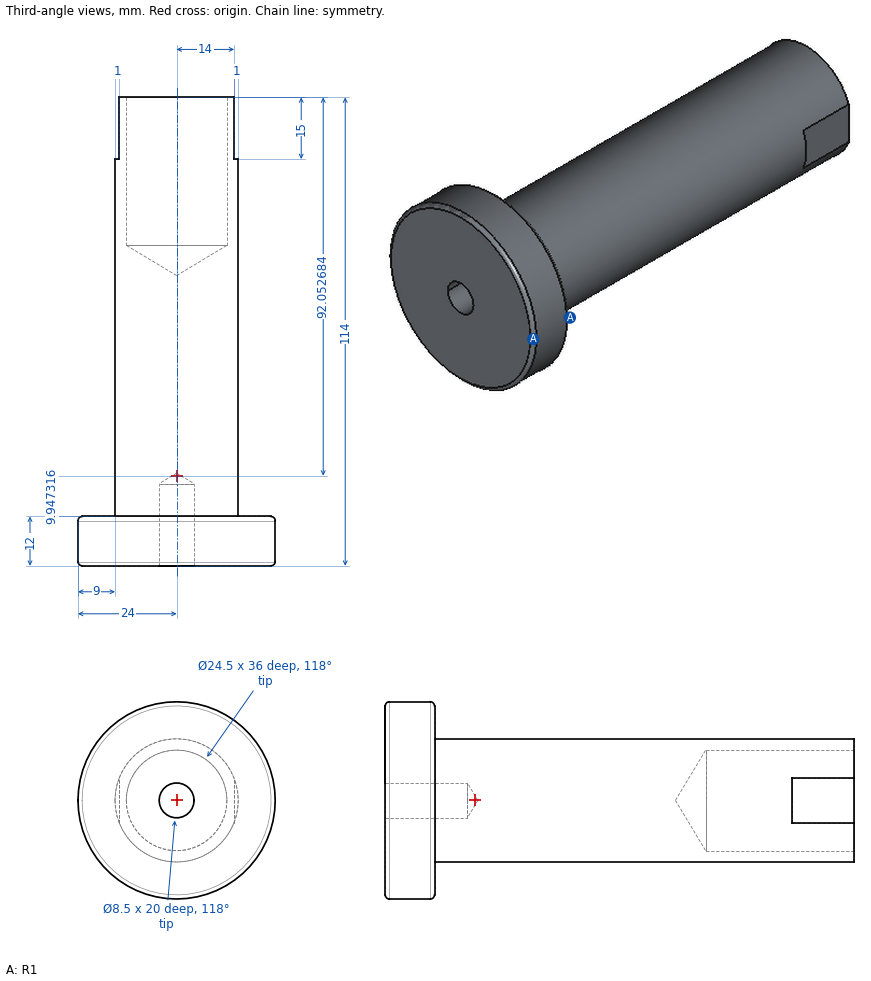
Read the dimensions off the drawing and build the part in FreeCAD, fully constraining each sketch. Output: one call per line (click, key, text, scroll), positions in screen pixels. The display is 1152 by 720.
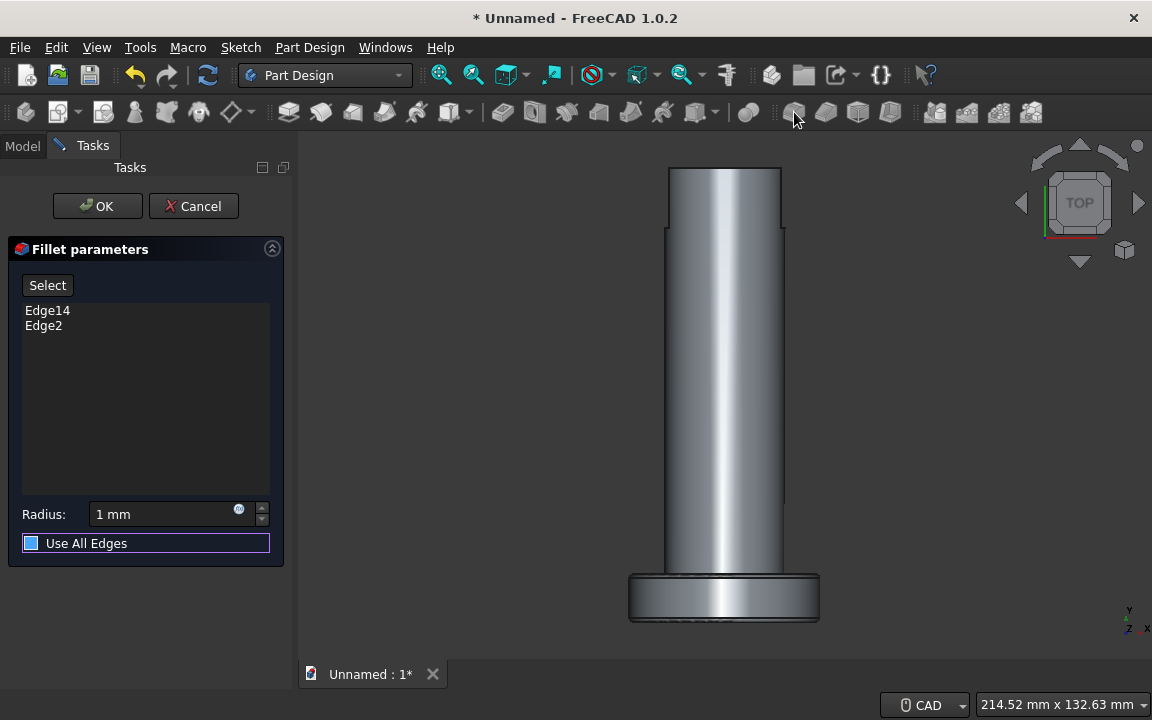
click(98, 206)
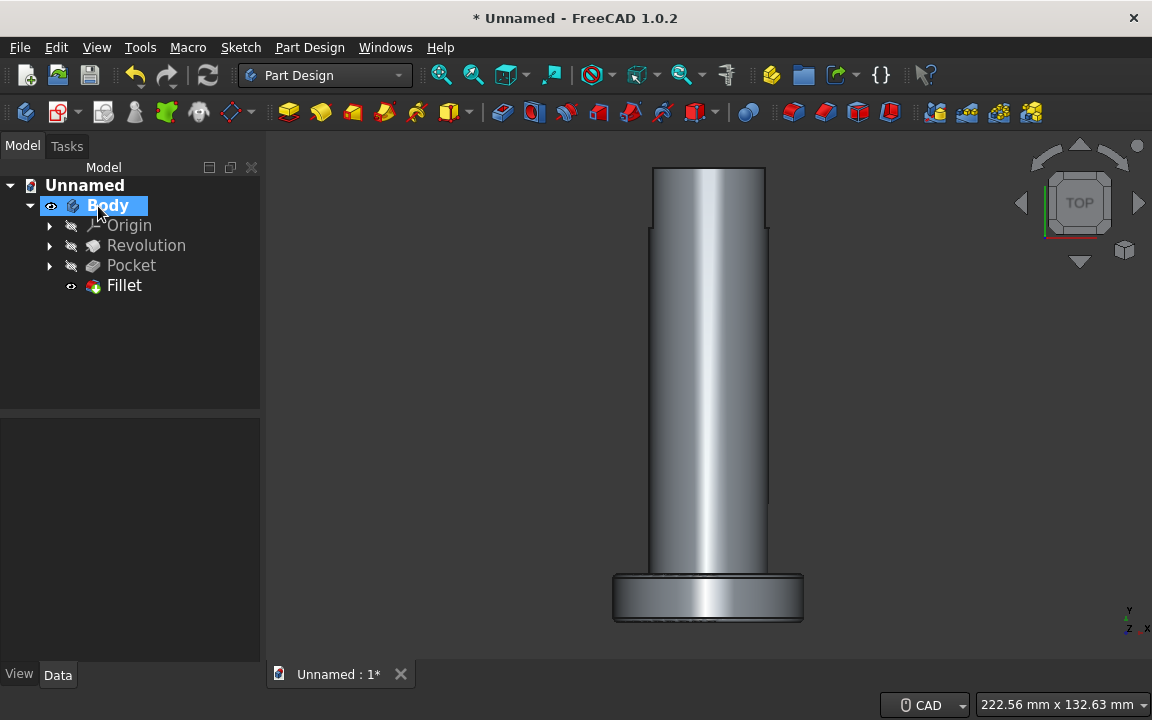
key(4)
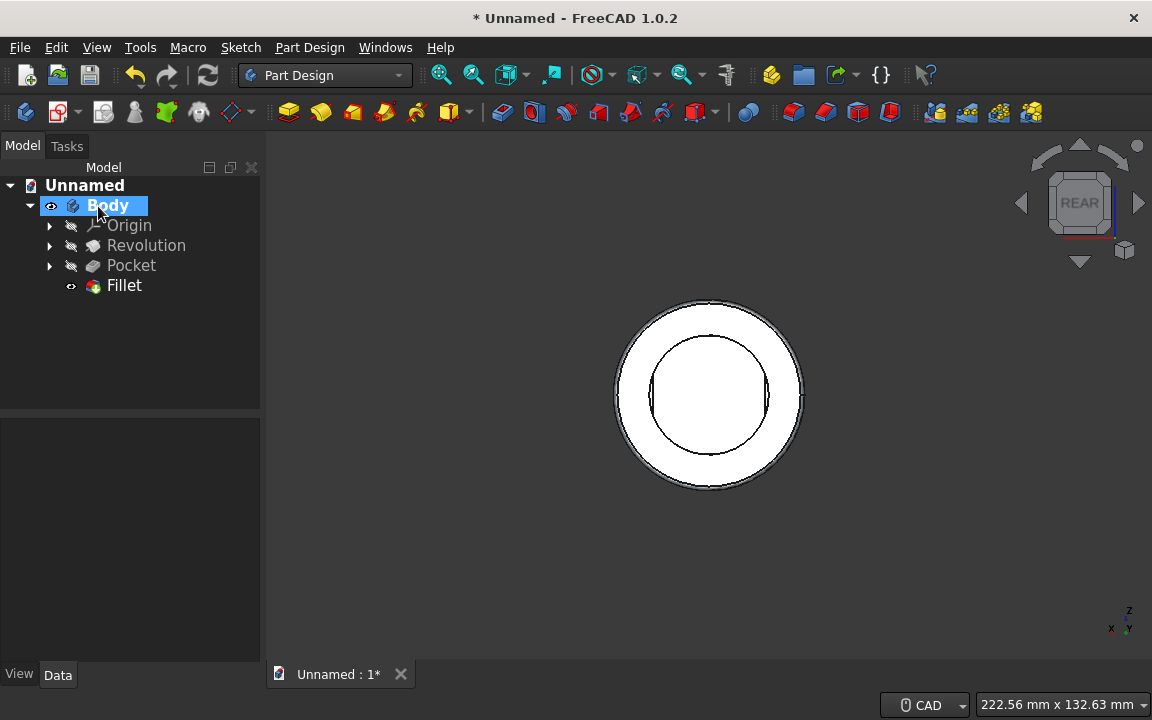
key(v)
key(f)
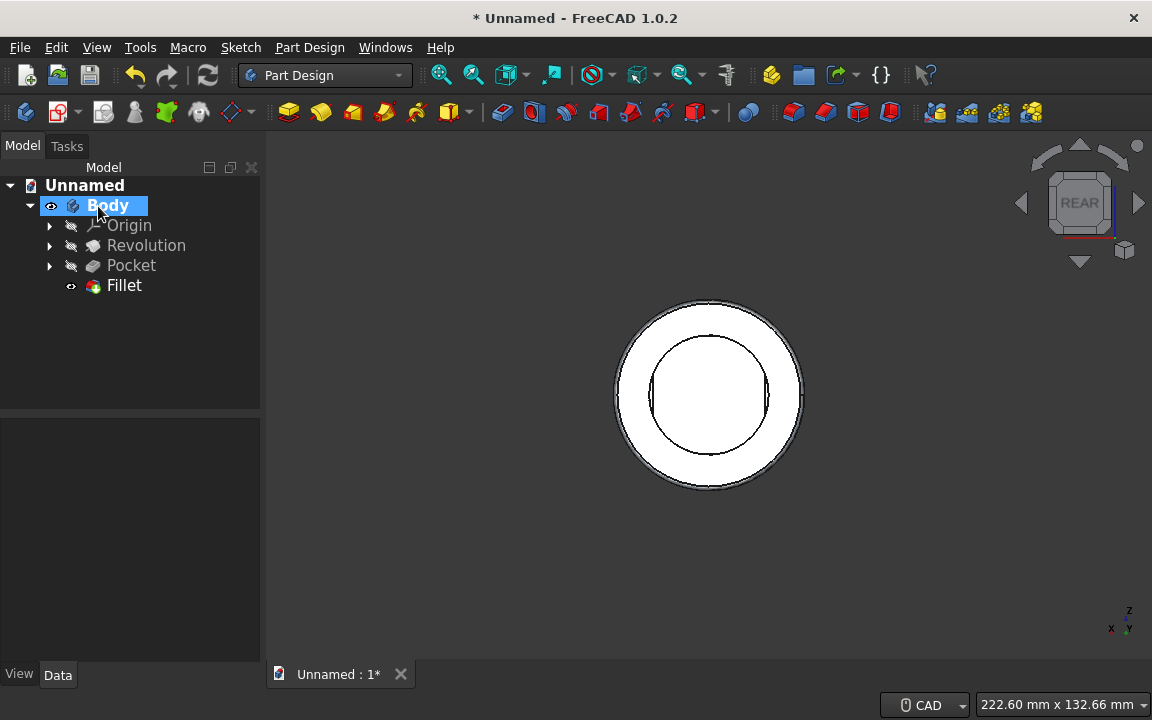
click(709, 394)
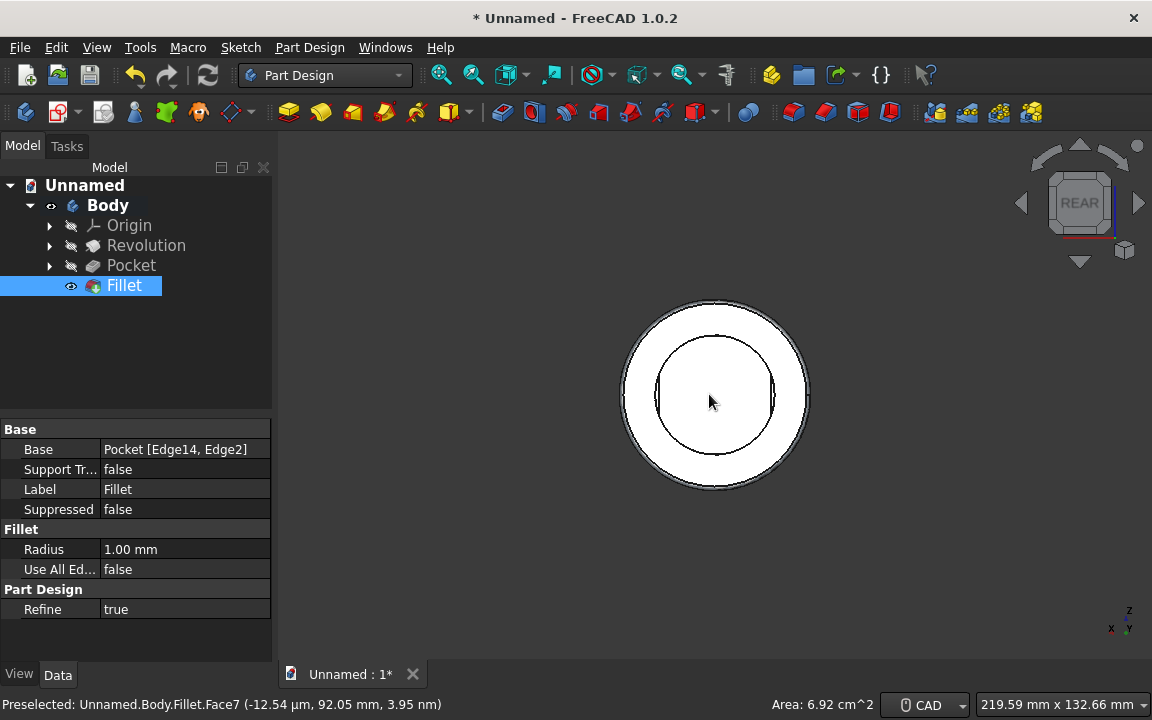
click(58, 112)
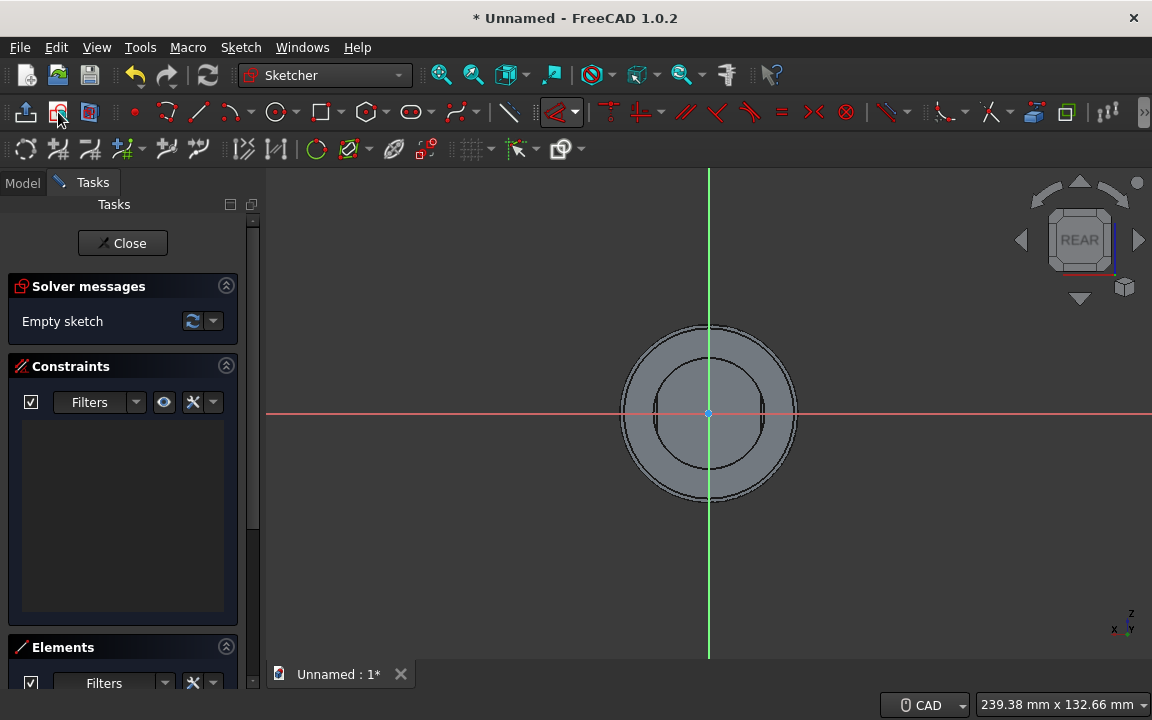
scroll(738, 414, up, 6)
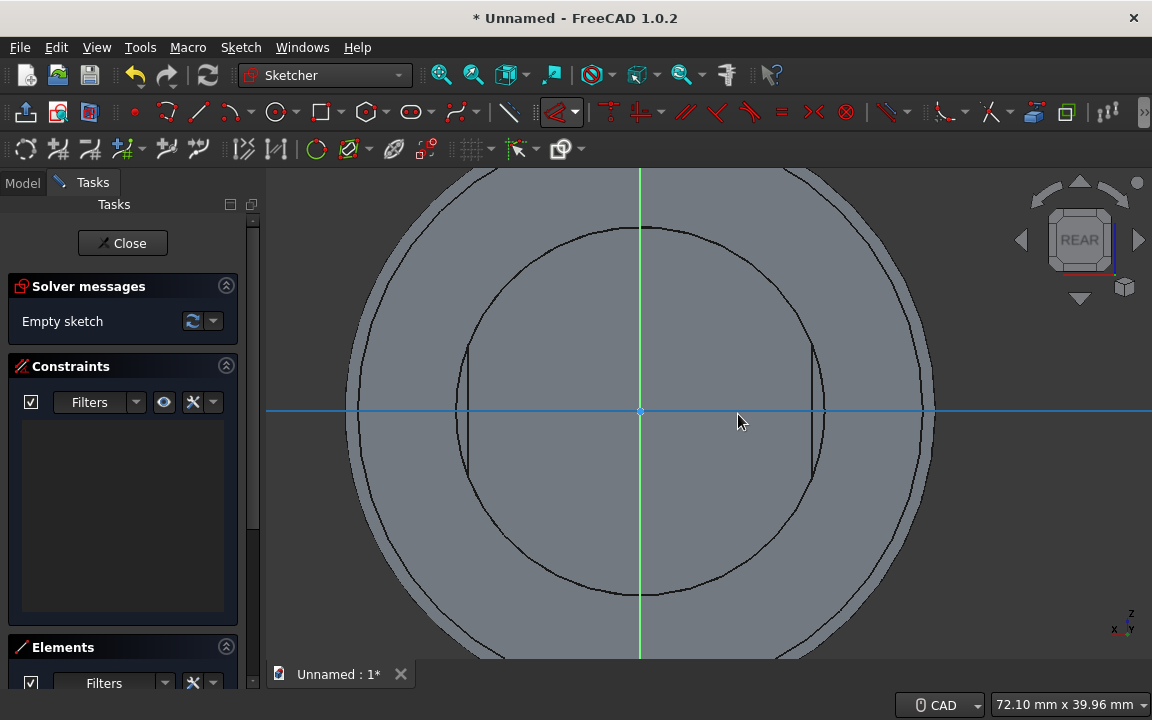
key(g)
key(c)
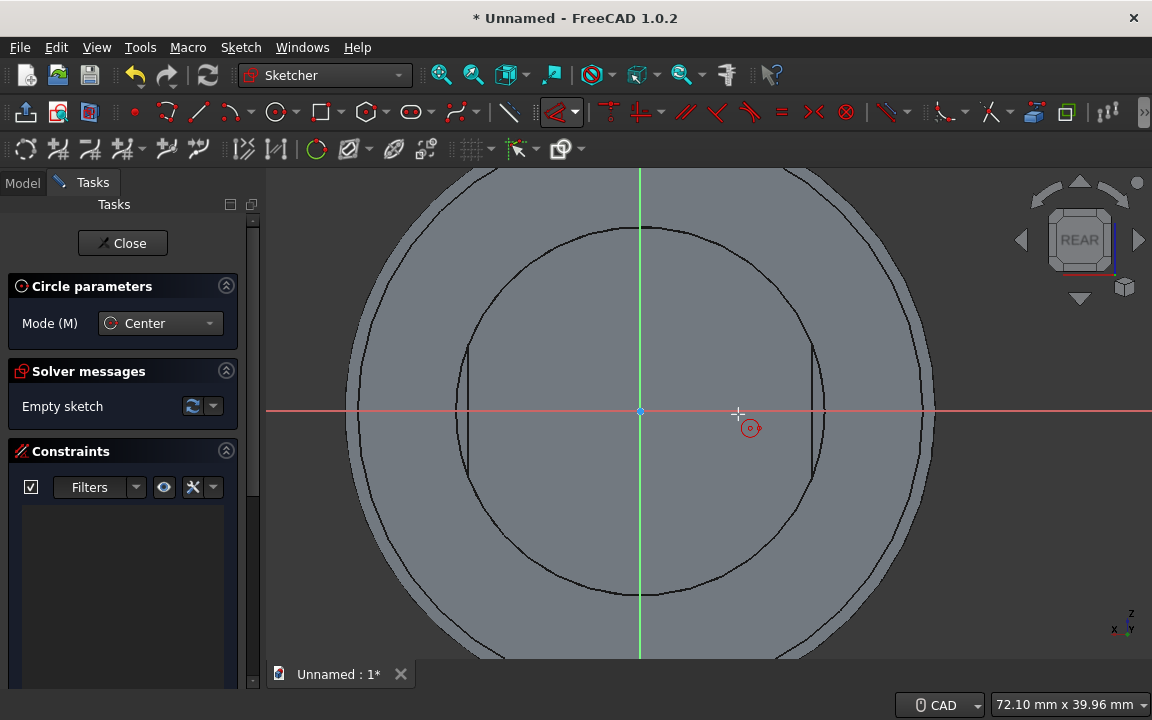
click(640, 411)
move(747, 305)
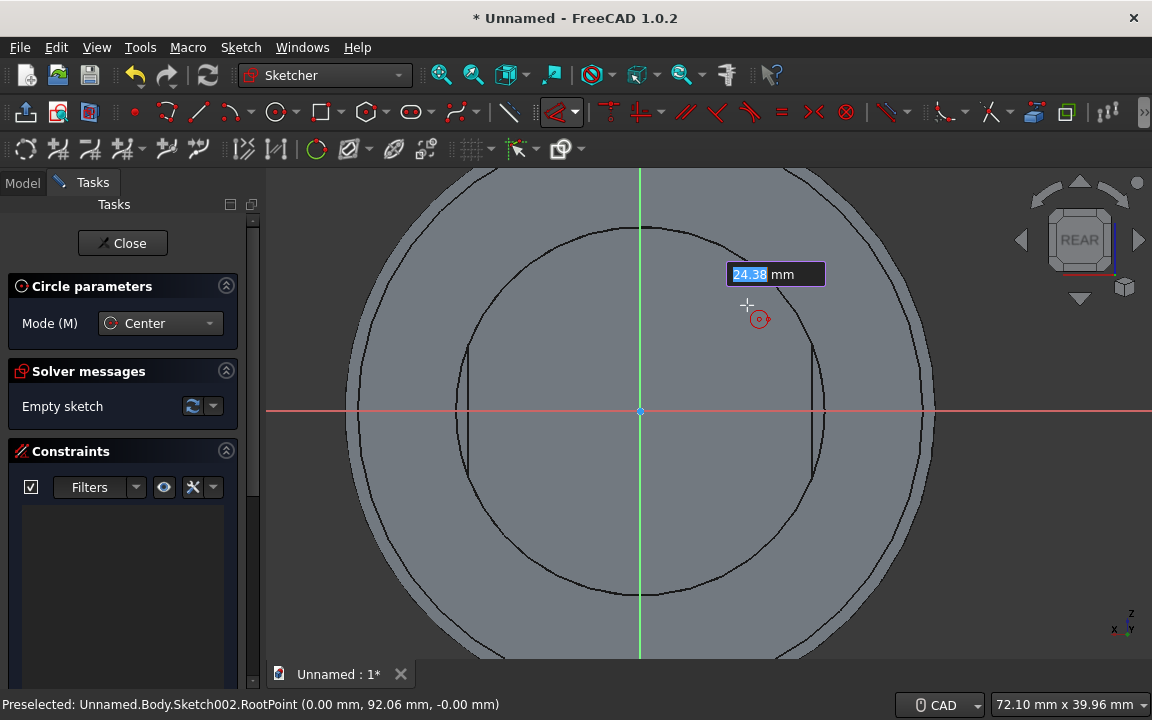
text(24.5)
key(Return)
key(Escape)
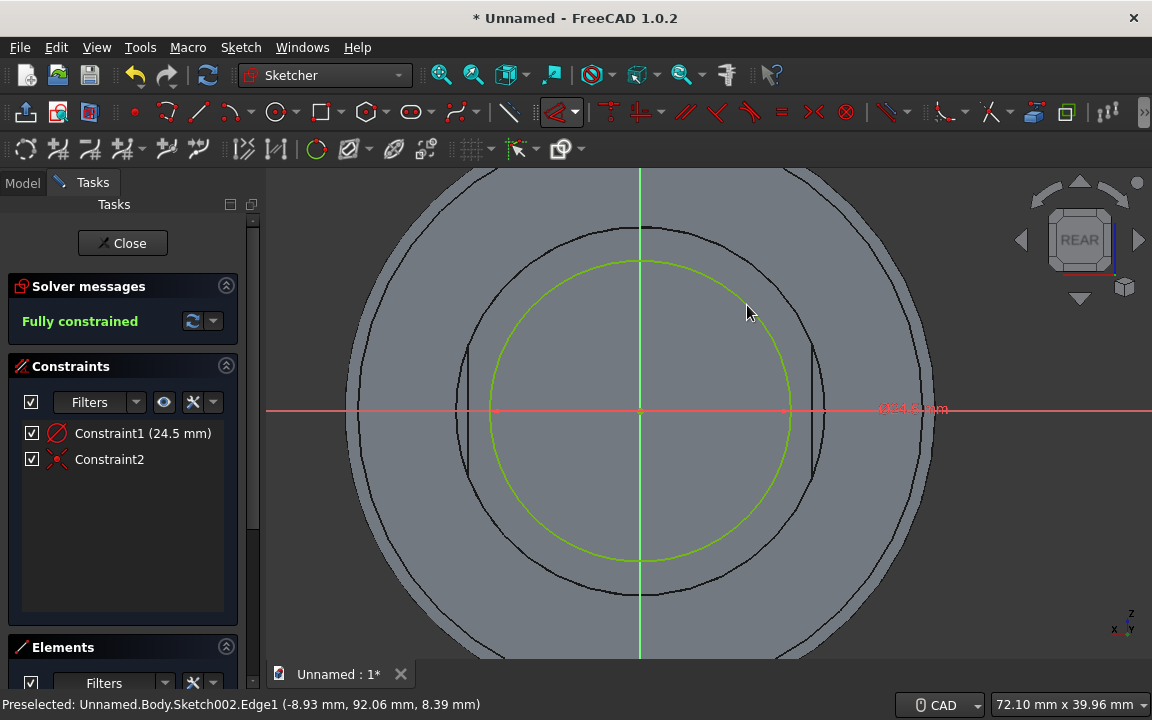
click(123, 243)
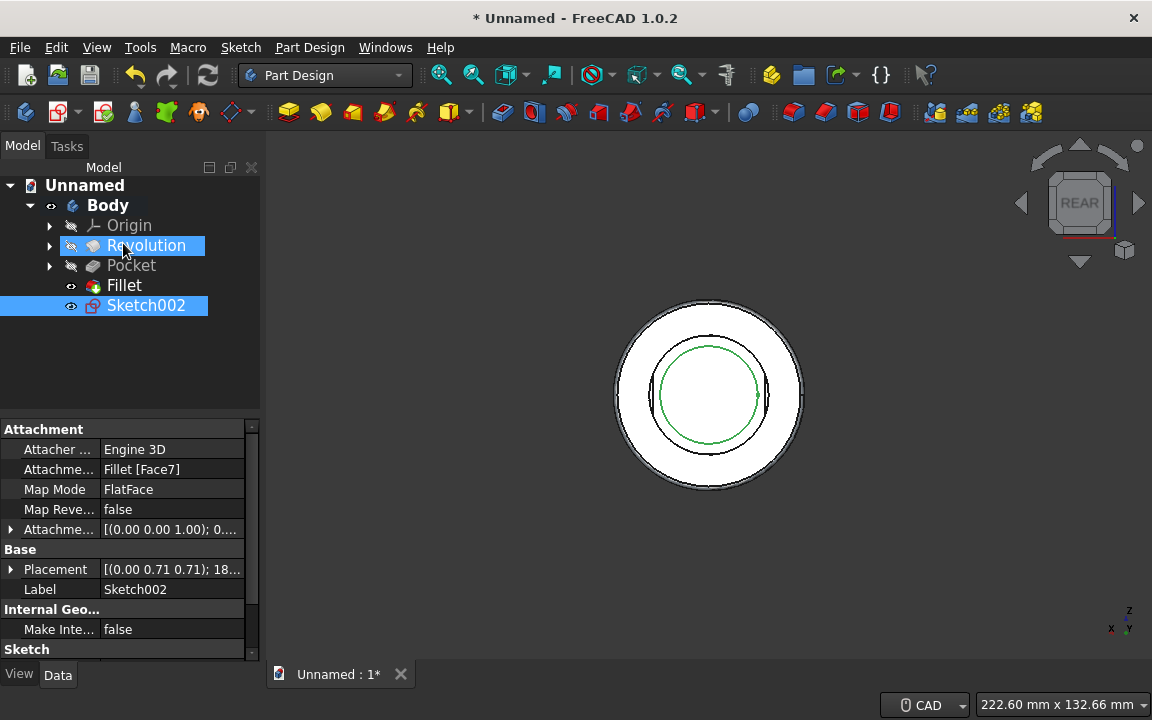
click(536, 112)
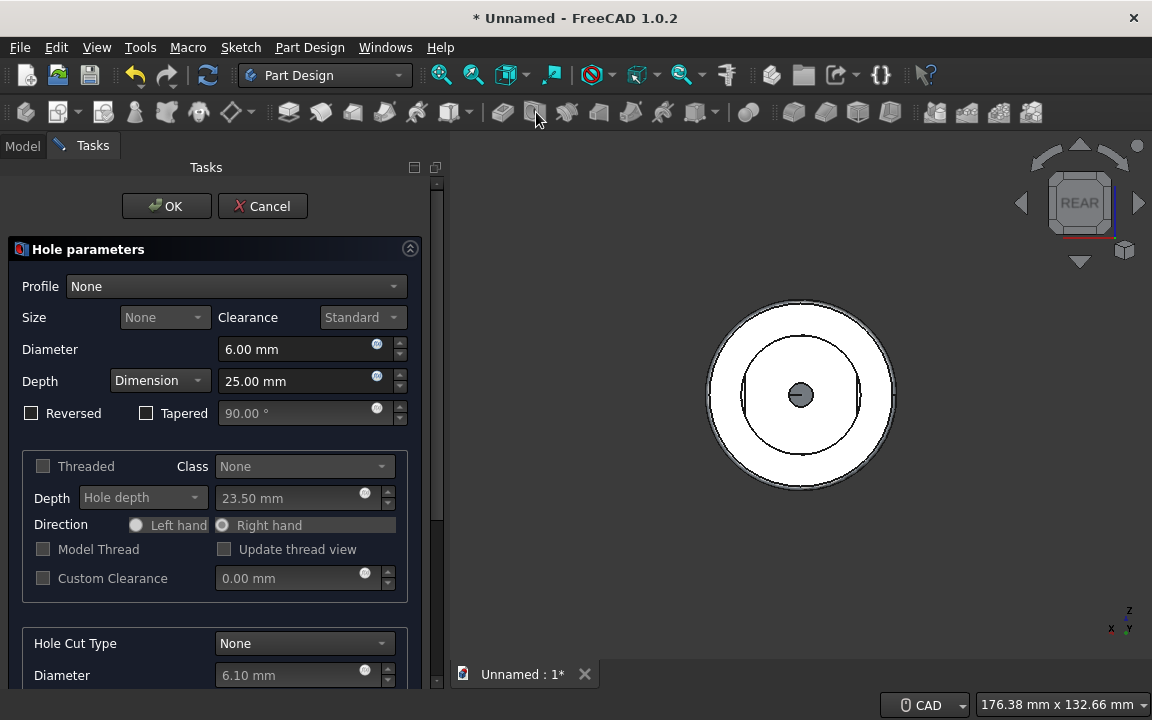
triple_click(305, 349)